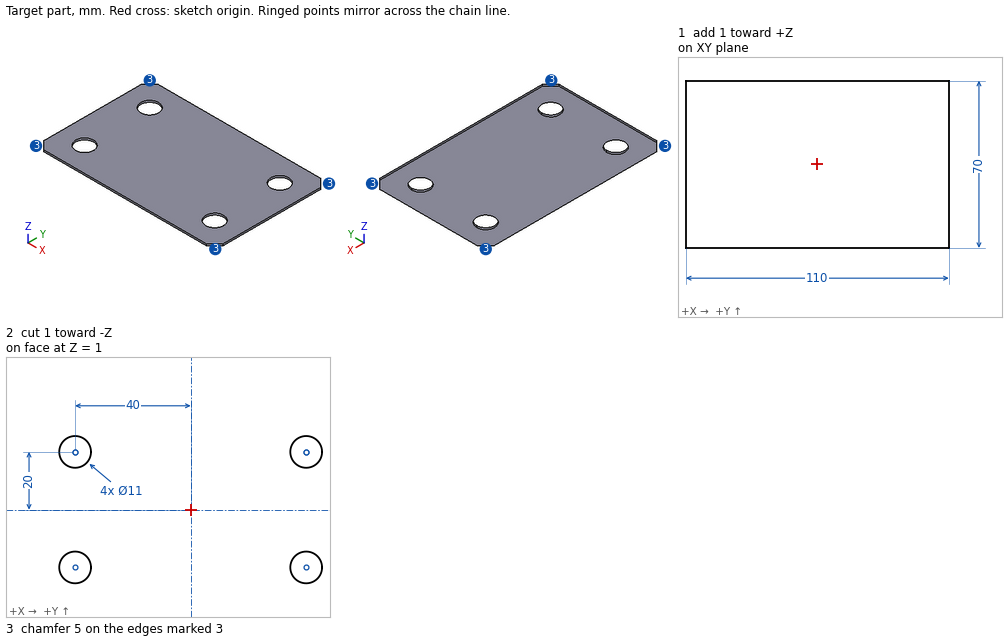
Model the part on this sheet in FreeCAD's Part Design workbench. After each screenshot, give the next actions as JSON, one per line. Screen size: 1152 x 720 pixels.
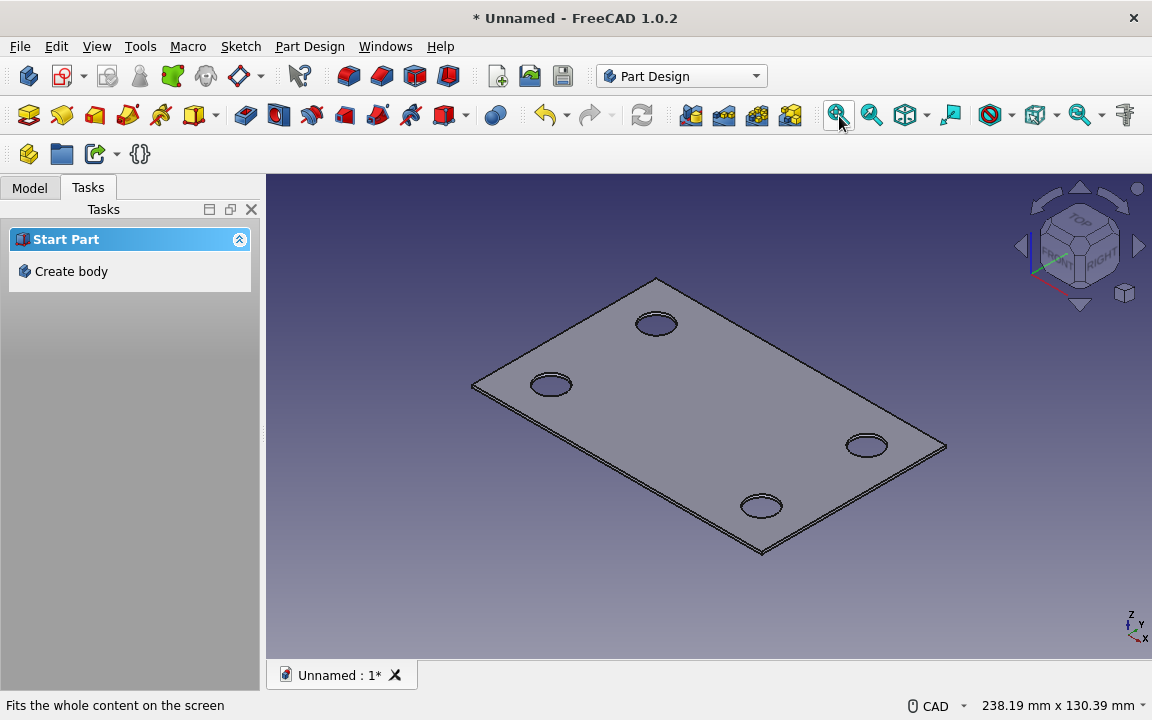
{"action": "key", "text": "2"}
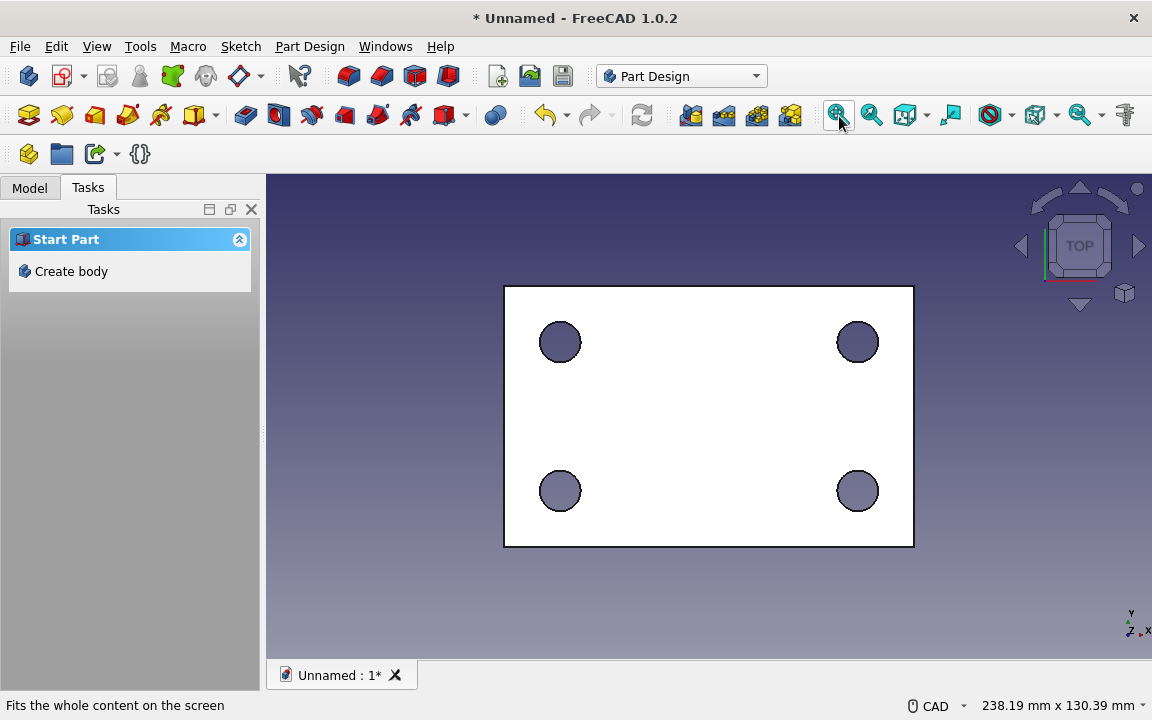
{"action": "scroll", "coordinate": [504, 285], "scroll_direction": "up", "scroll_amount": 12}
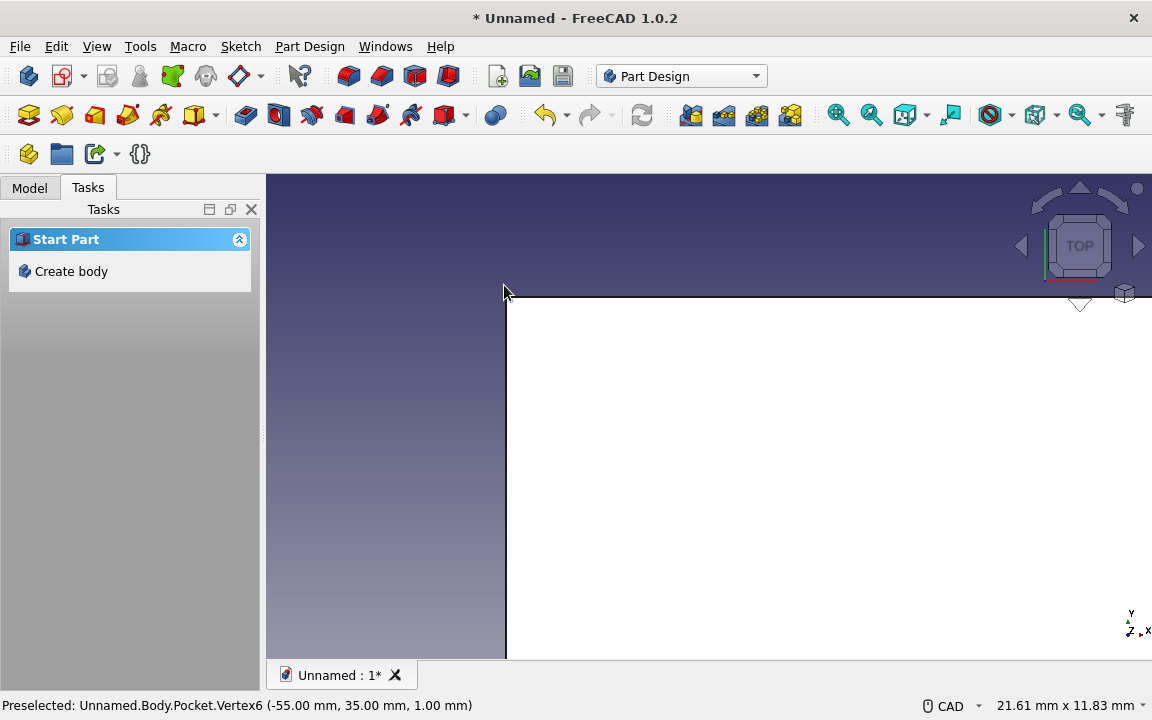
{"action": "left_click", "coordinate": [839, 116]}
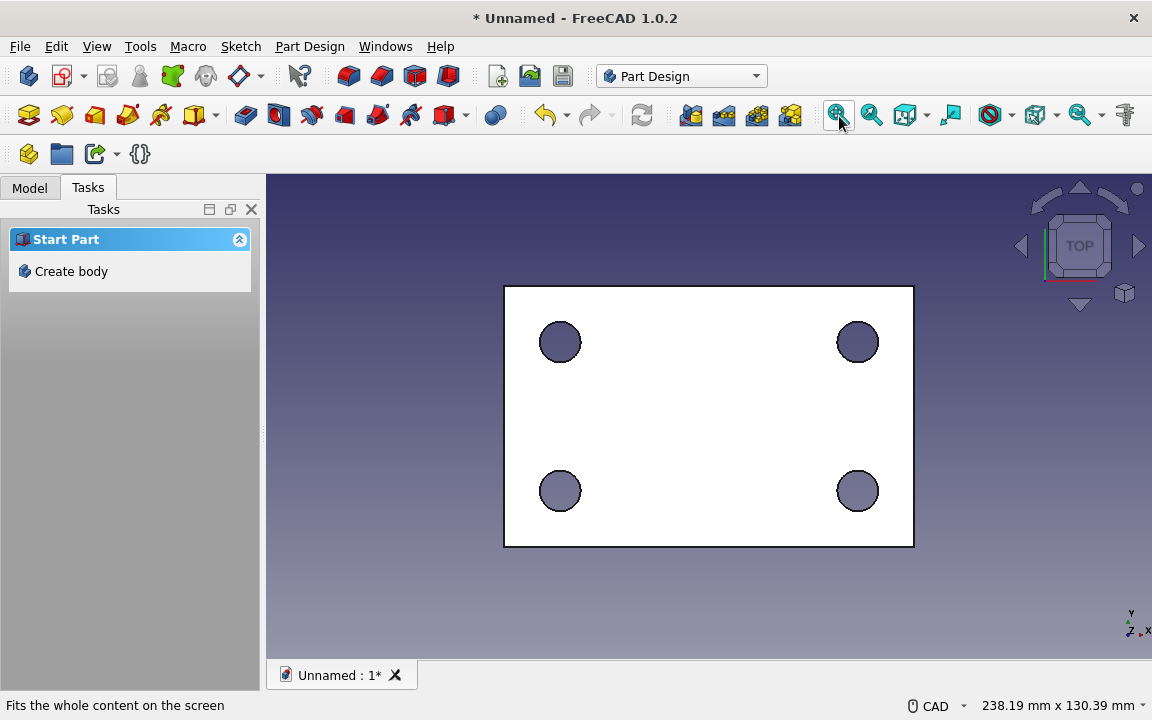
{"action": "key", "text": "1"}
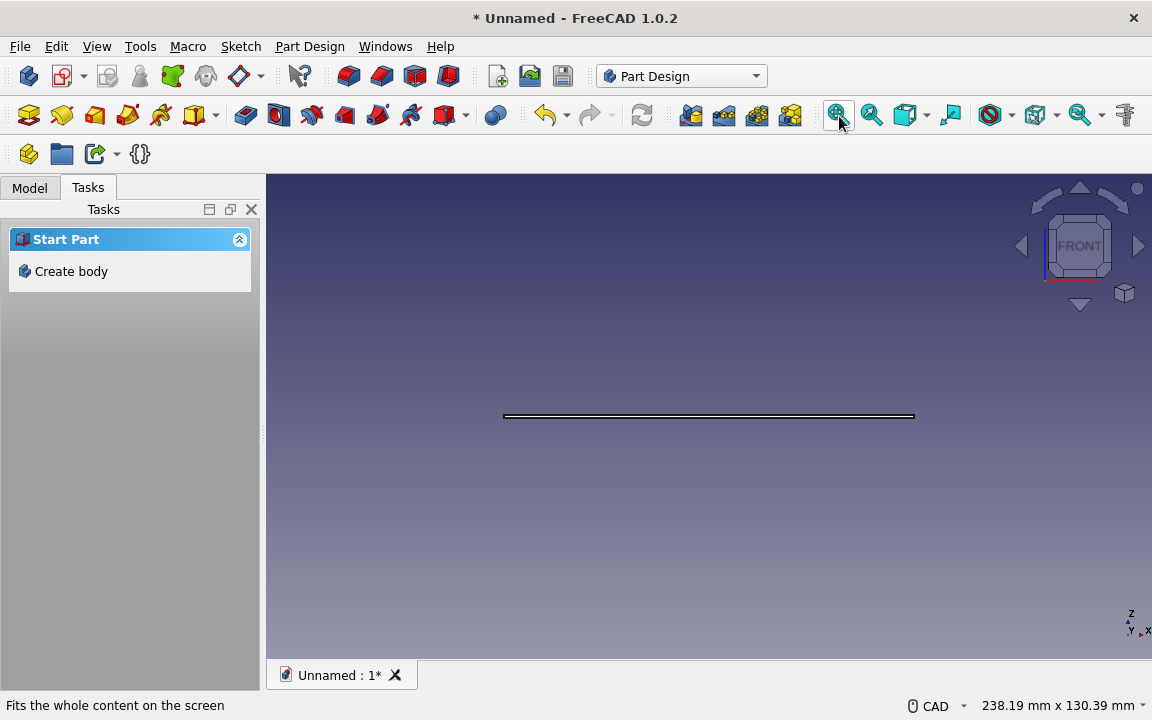
{"action": "scroll", "coordinate": [504, 415], "scroll_direction": "up", "scroll_amount": 12}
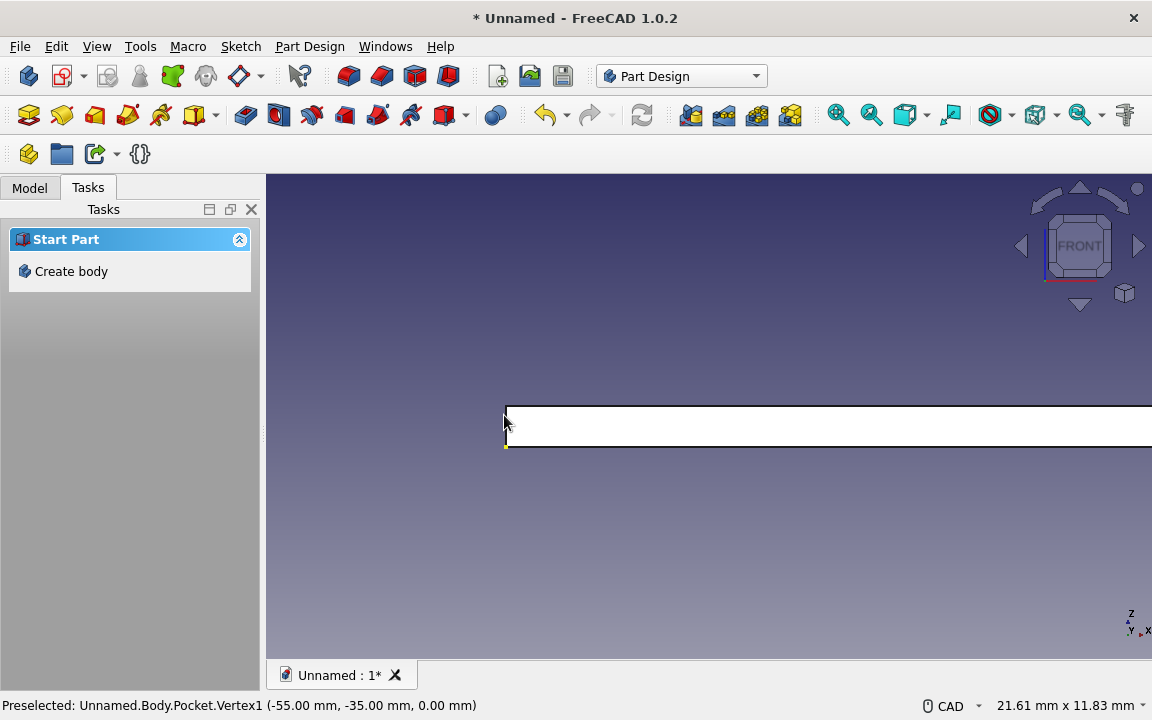
{"action": "left_click", "coordinate": [506, 426]}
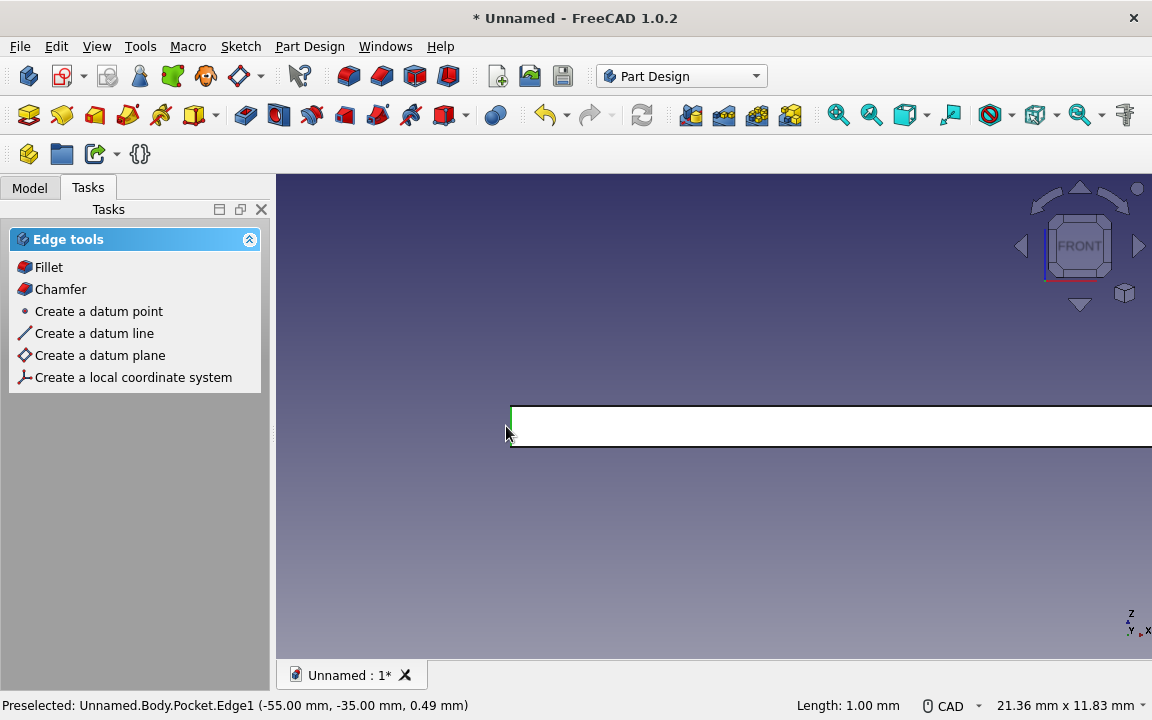
{"action": "left_click", "coordinate": [839, 116]}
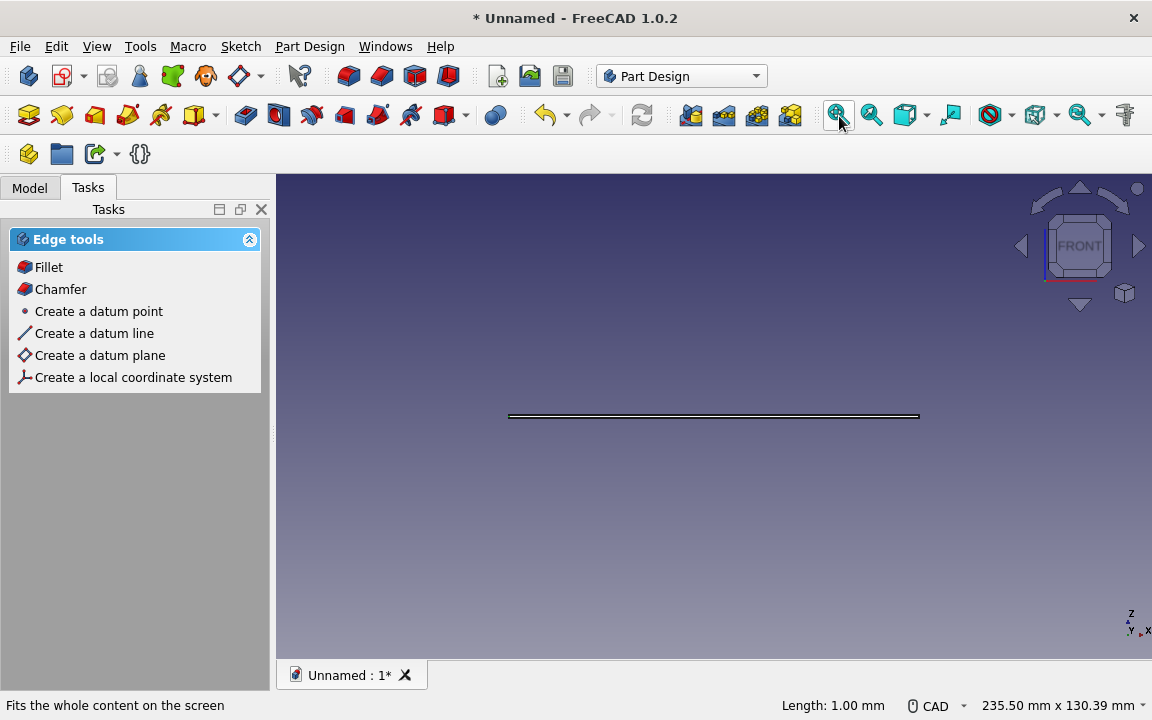
{"action": "key", "text": "3"}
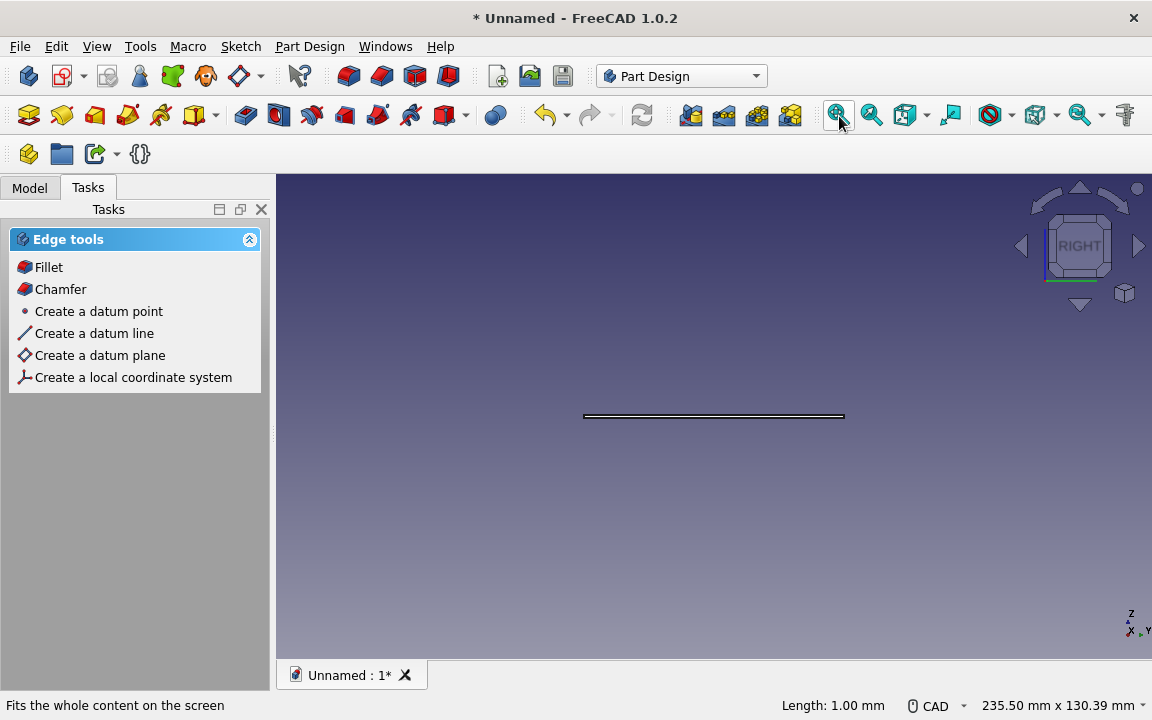
{"action": "left_click", "coordinate": [839, 116]}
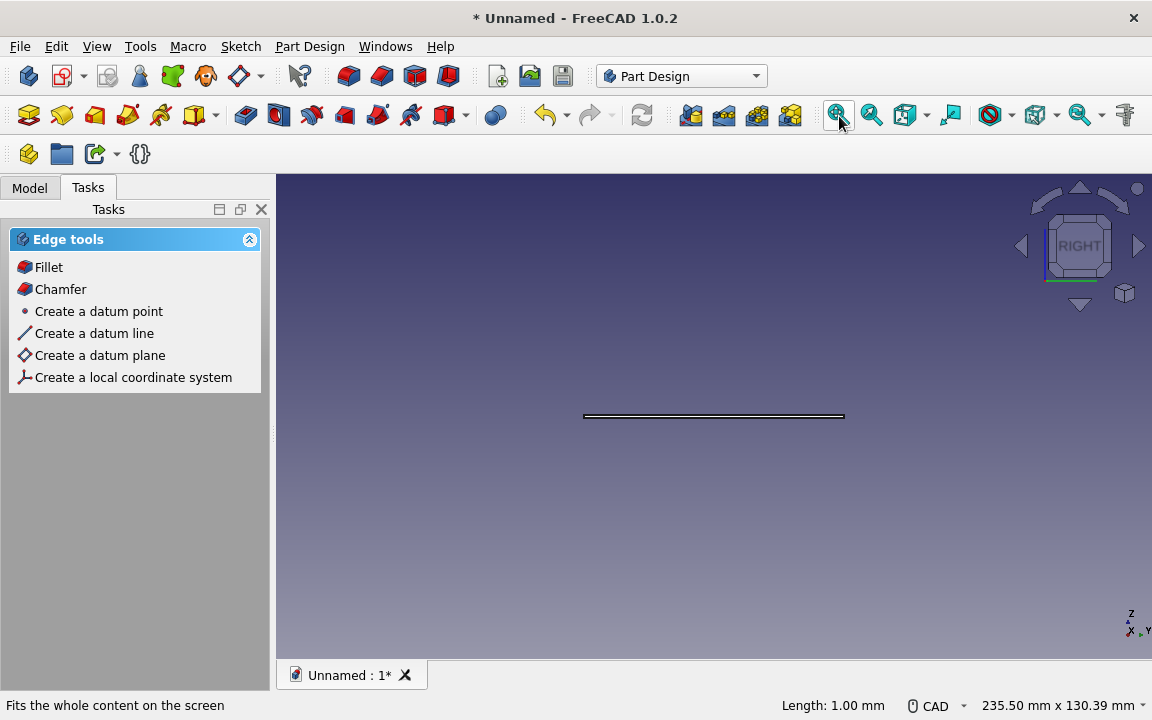
{"action": "scroll", "coordinate": [844, 415], "scroll_direction": "up", "scroll_amount": 12}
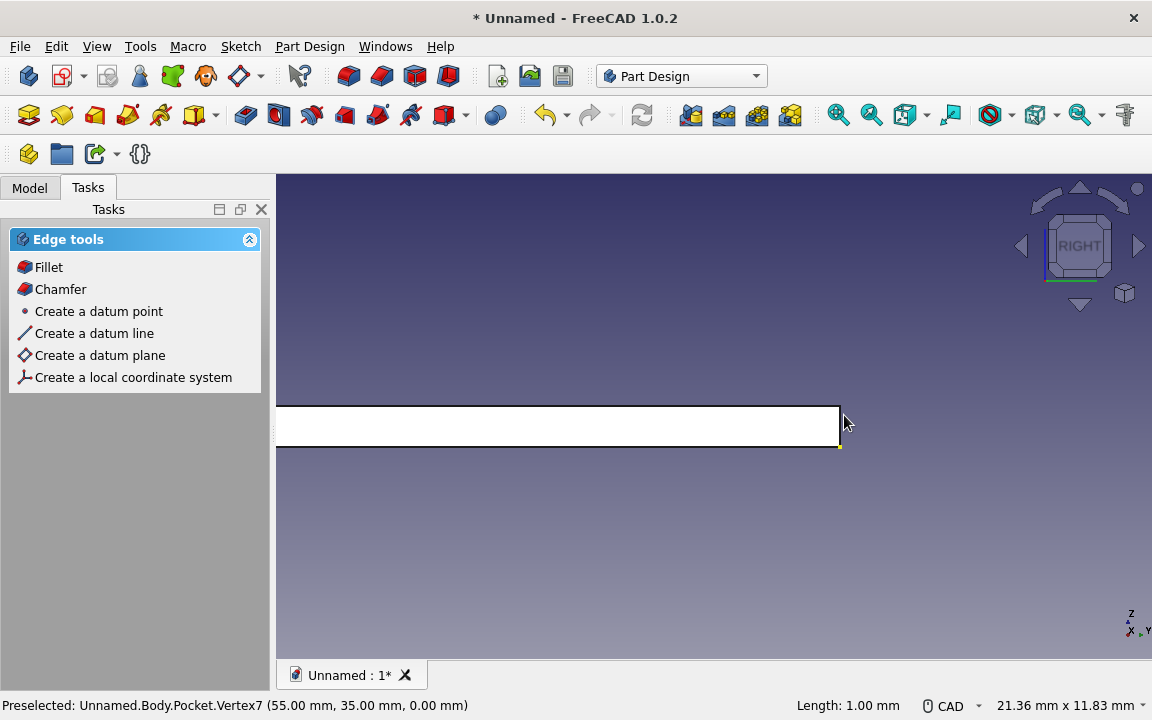
{"action": "left_click", "coordinate": [840, 426], "text": "ctrl"}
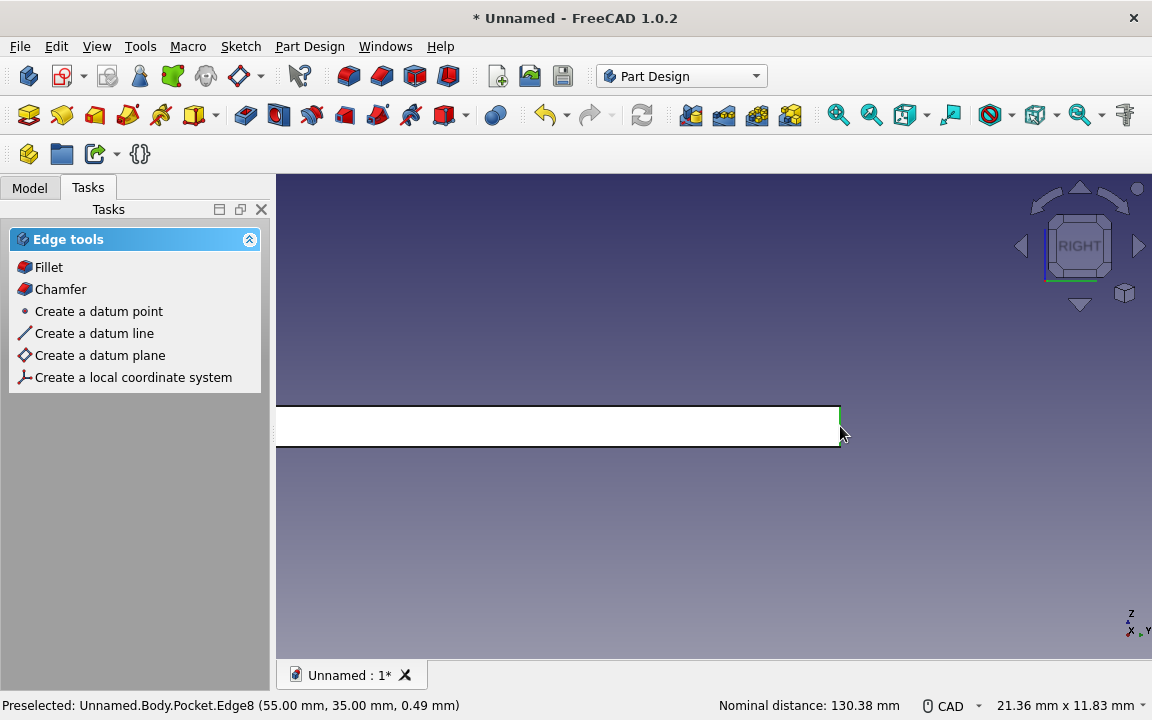
{"action": "left_click", "coordinate": [839, 116]}